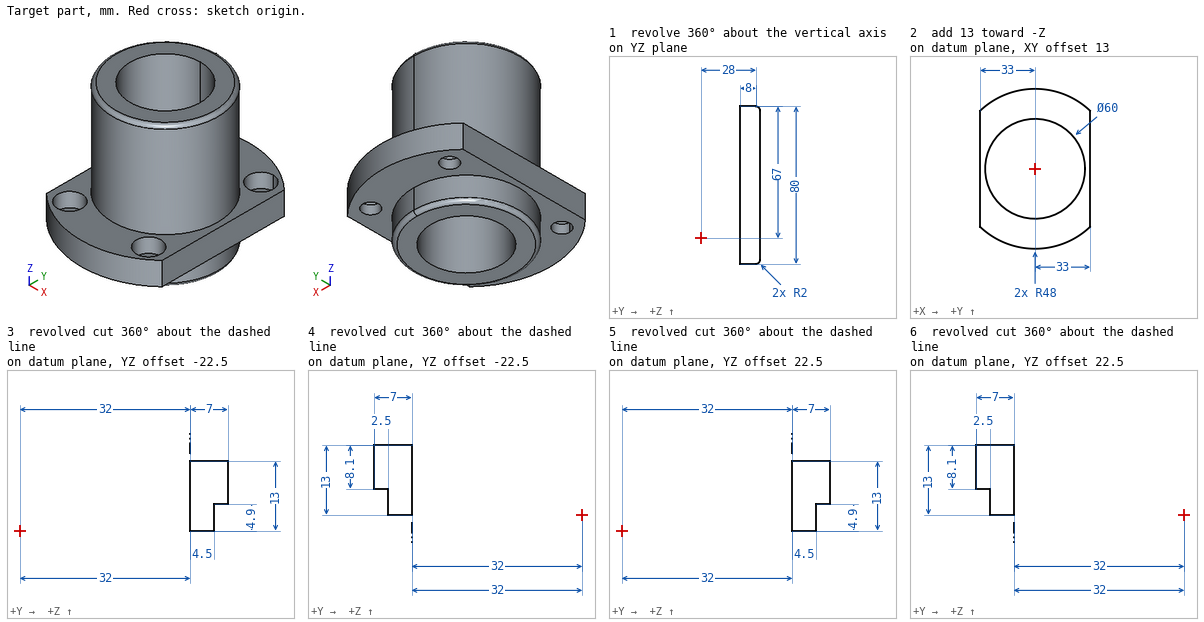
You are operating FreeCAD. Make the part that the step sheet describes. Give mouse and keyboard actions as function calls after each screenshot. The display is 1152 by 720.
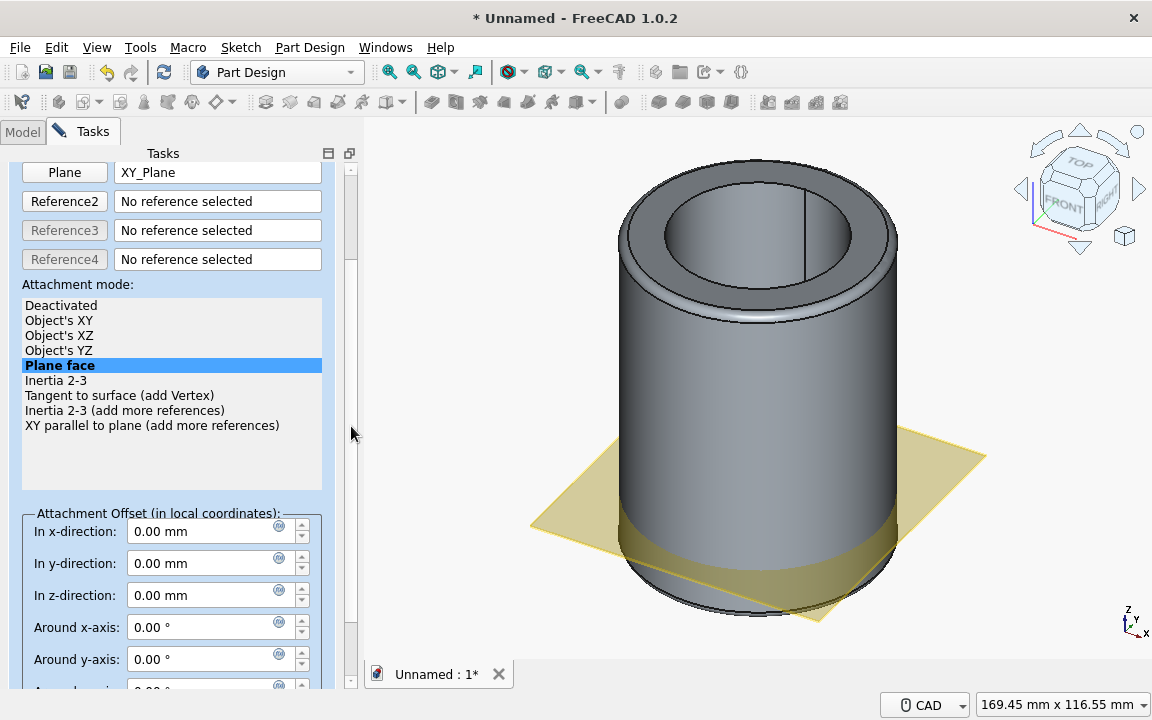
triple_click(210, 595)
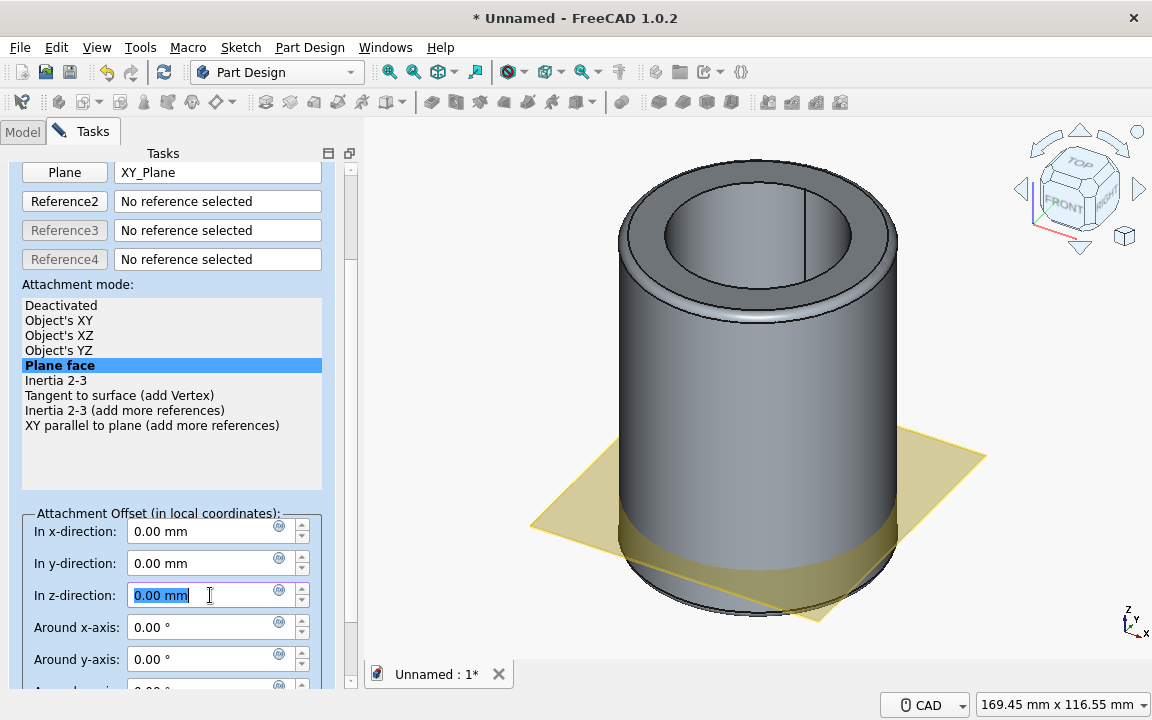
text(13)
key(Tab)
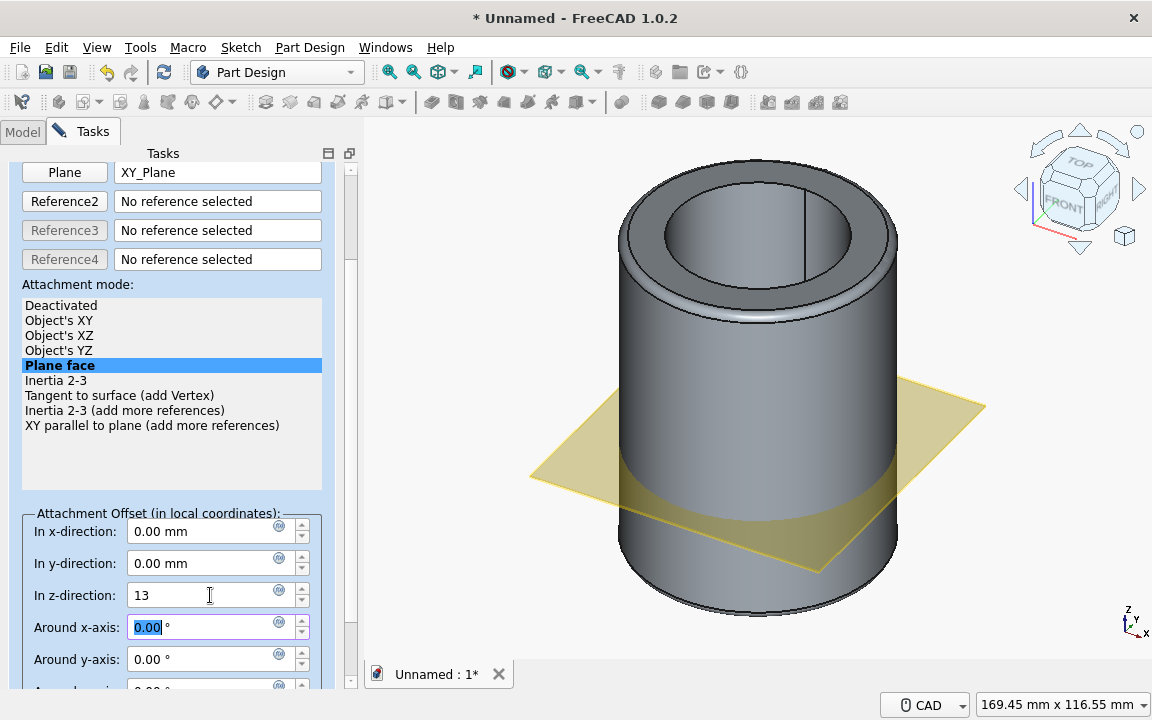
scroll(351, 426, up, 3)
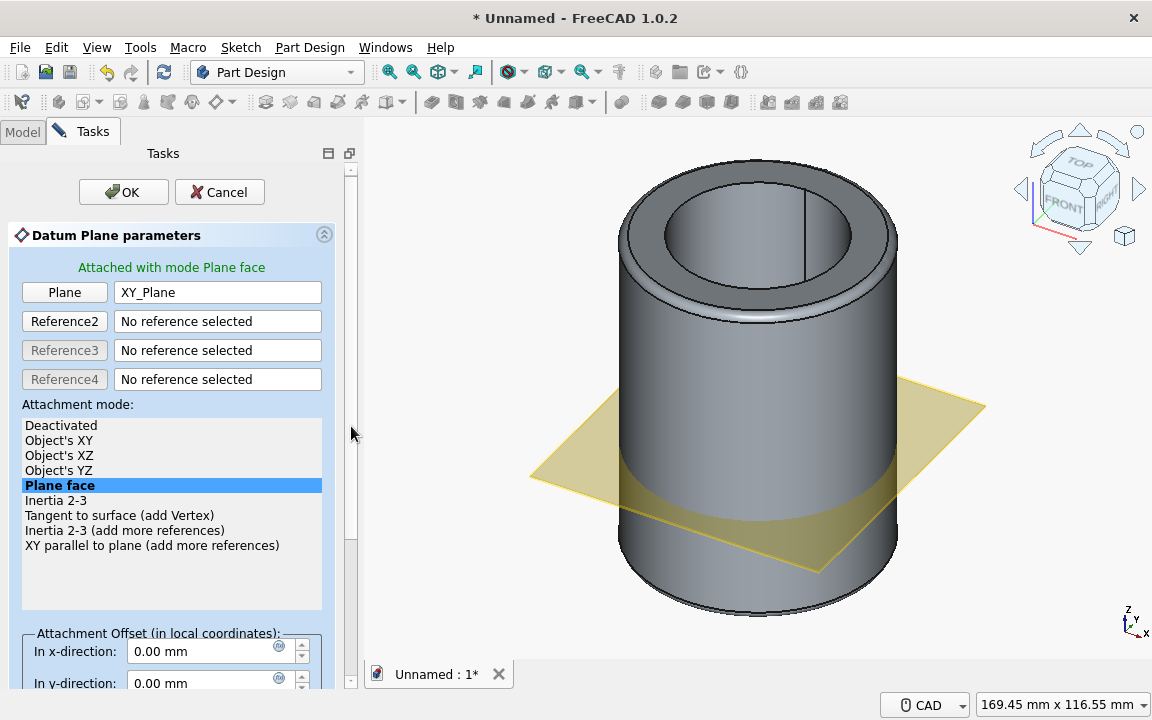
click(124, 192)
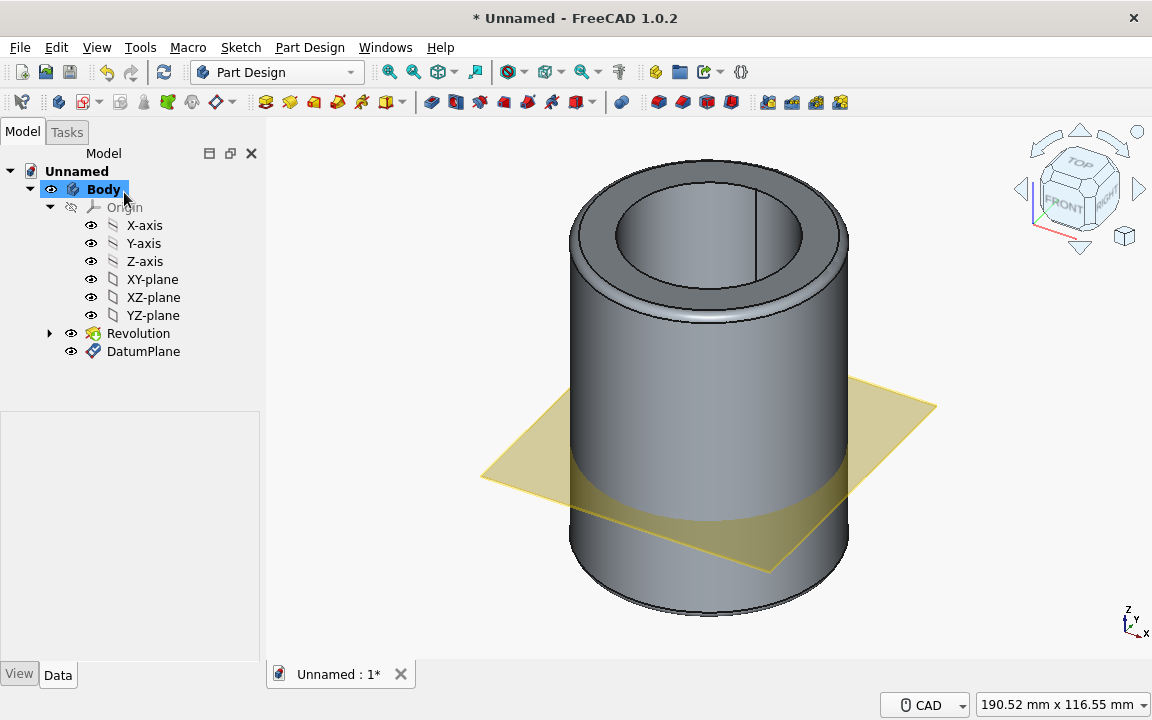
click(116, 351)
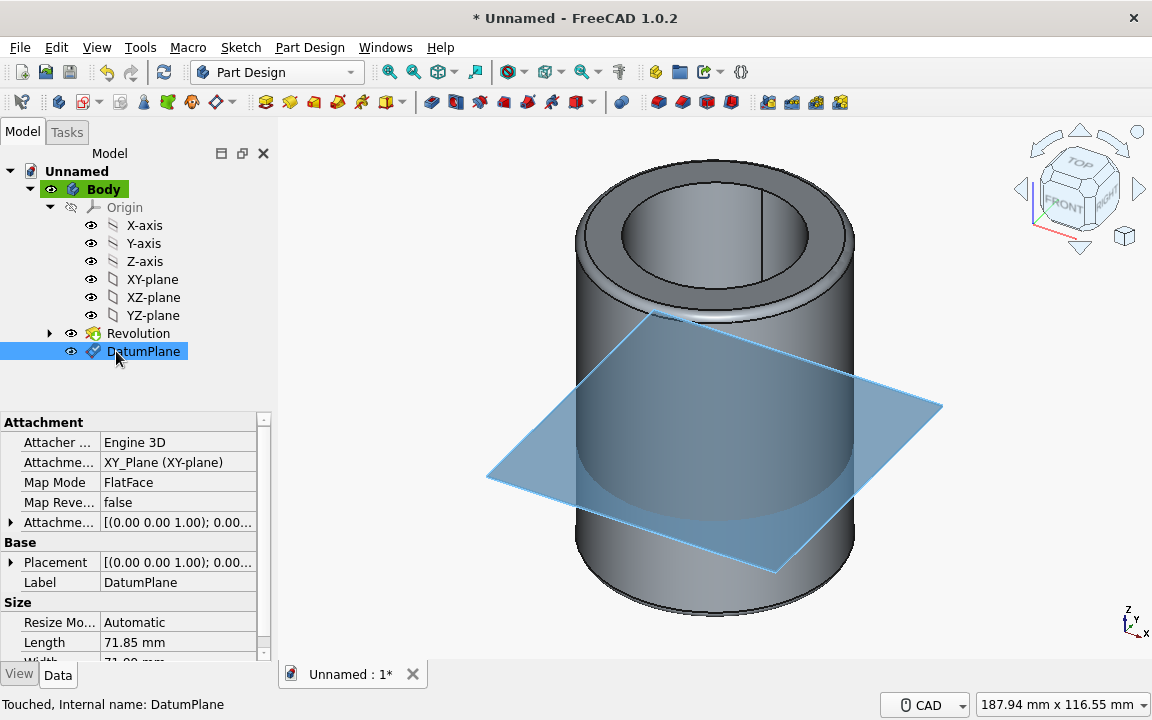
click(84, 102)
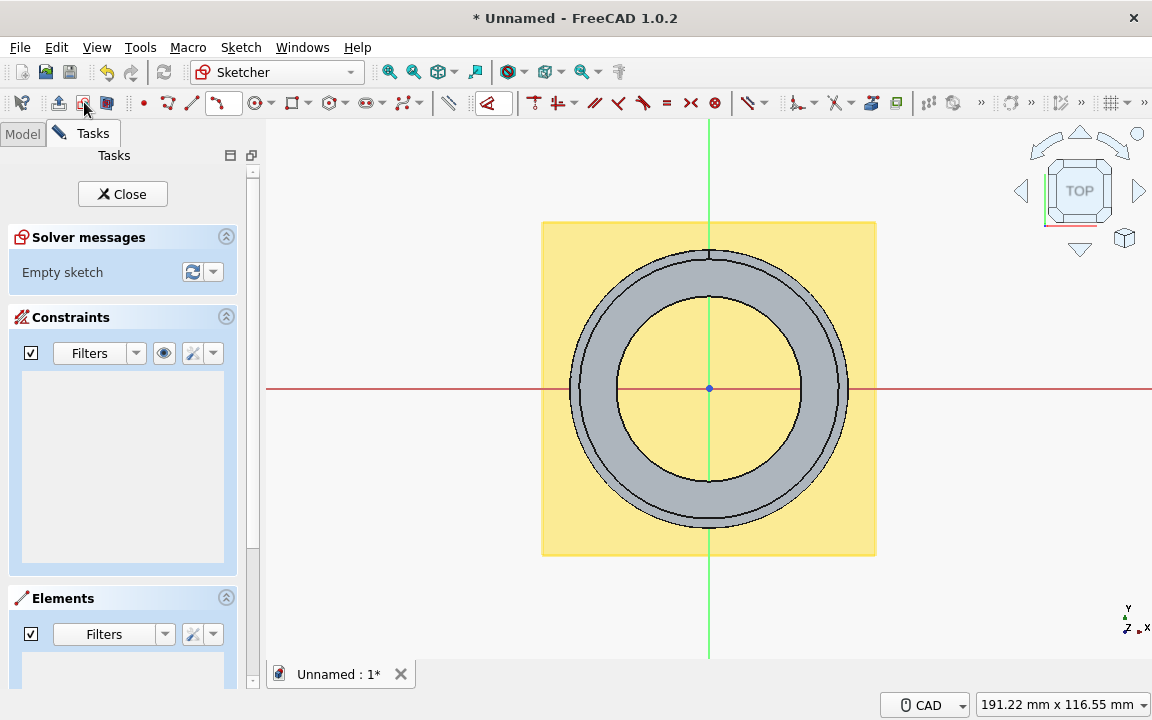
click(108, 104)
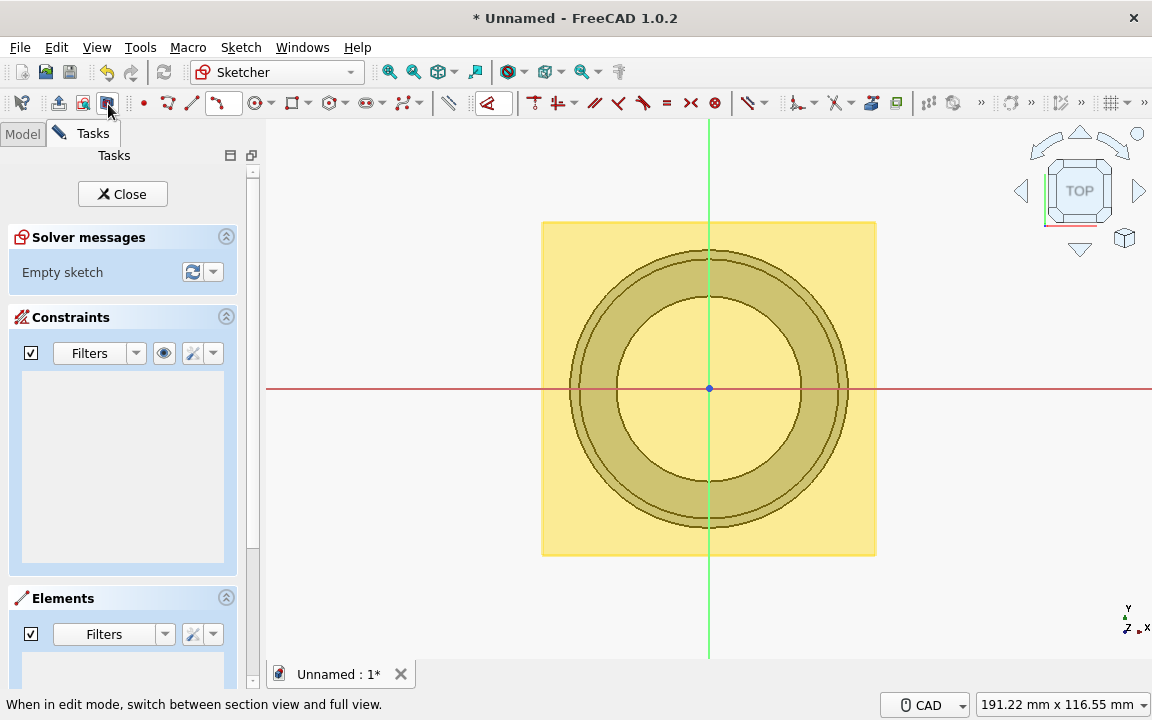
scroll(331, 389, down, 1)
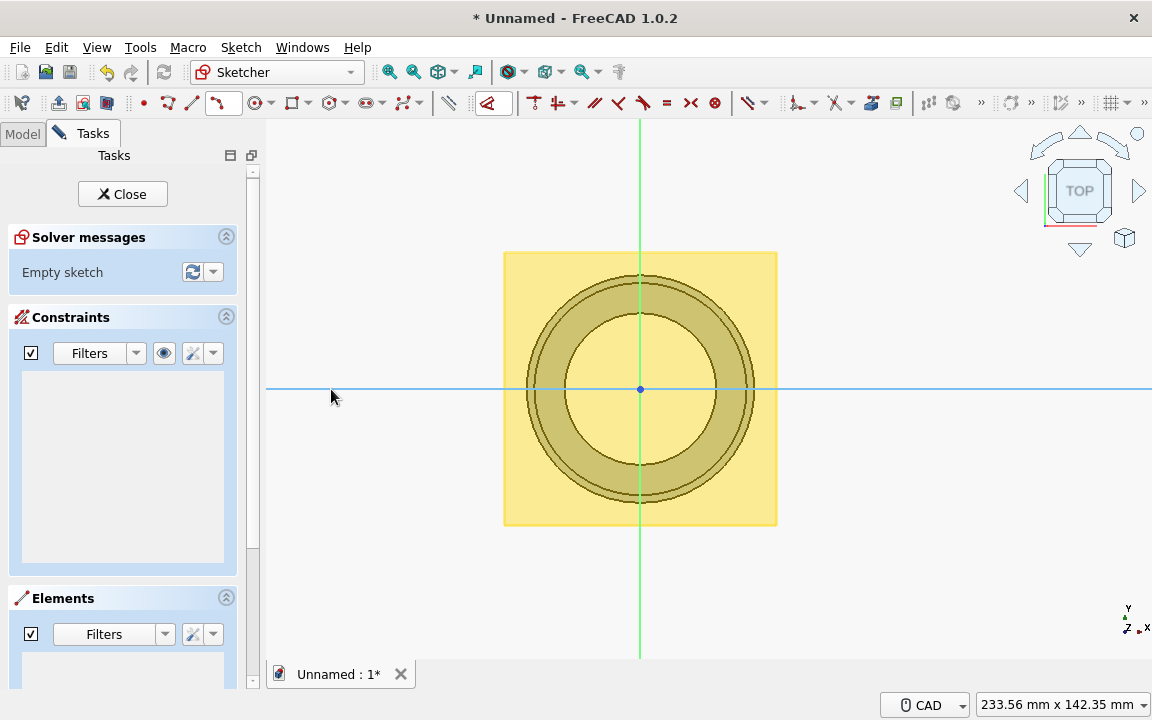
click(192, 104)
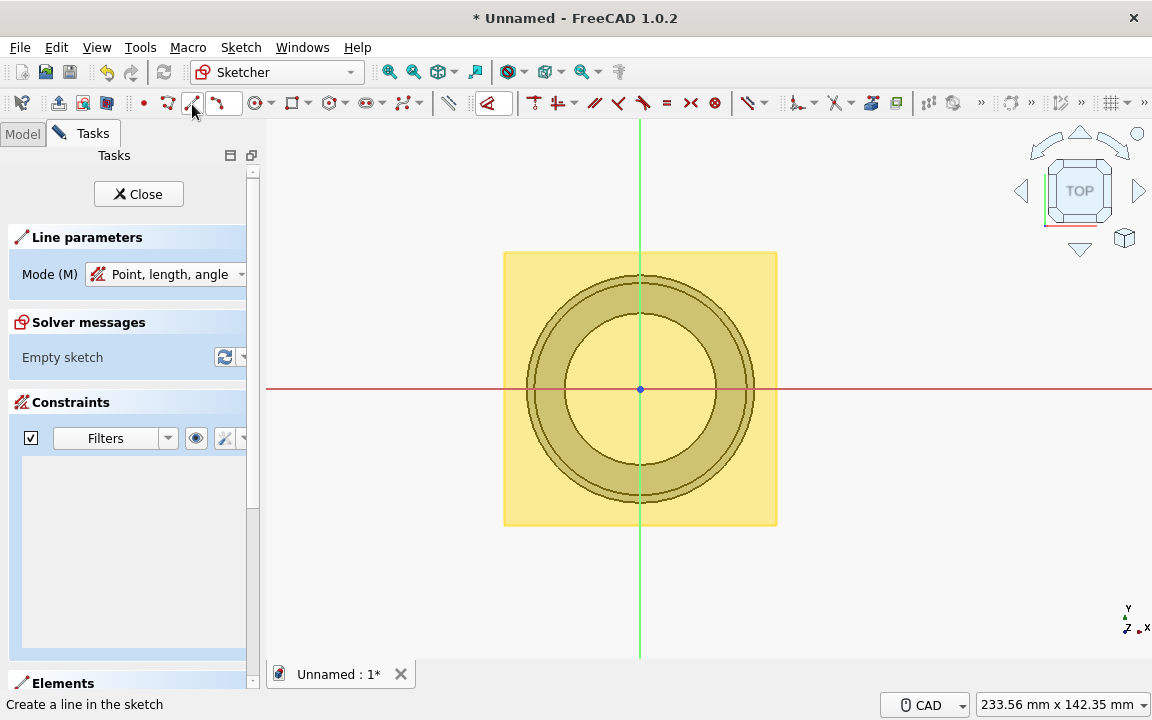
click(515, 257)
click(515, 521)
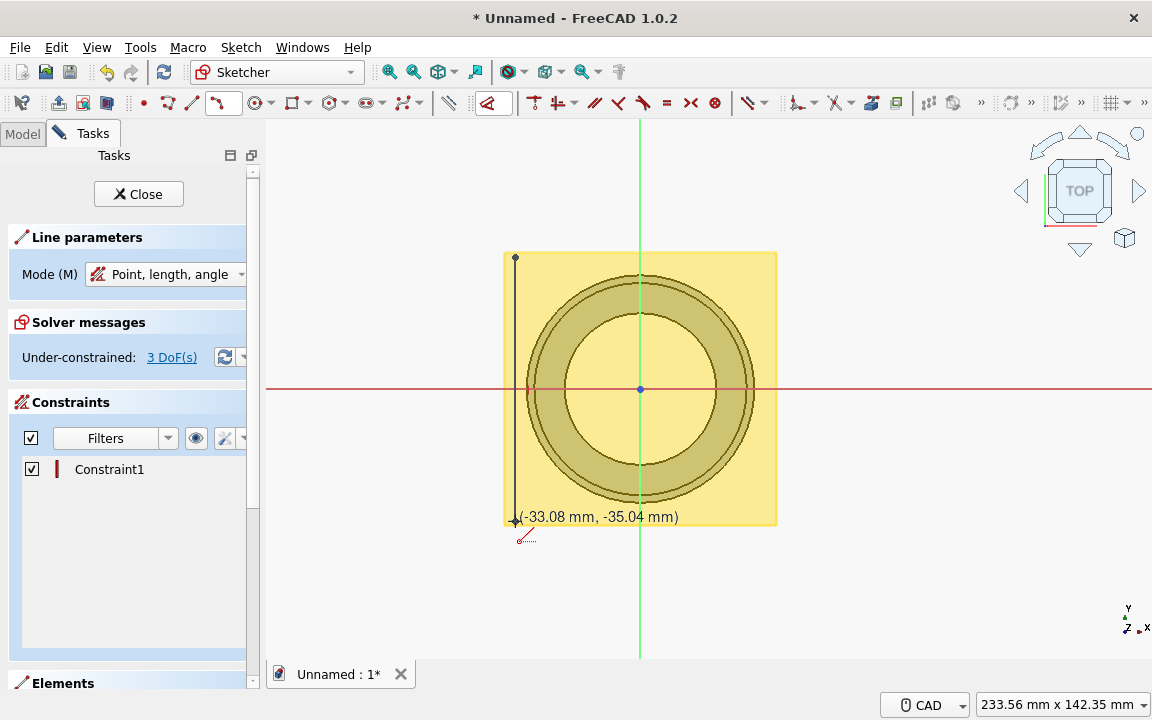
click(766, 521)
click(766, 257)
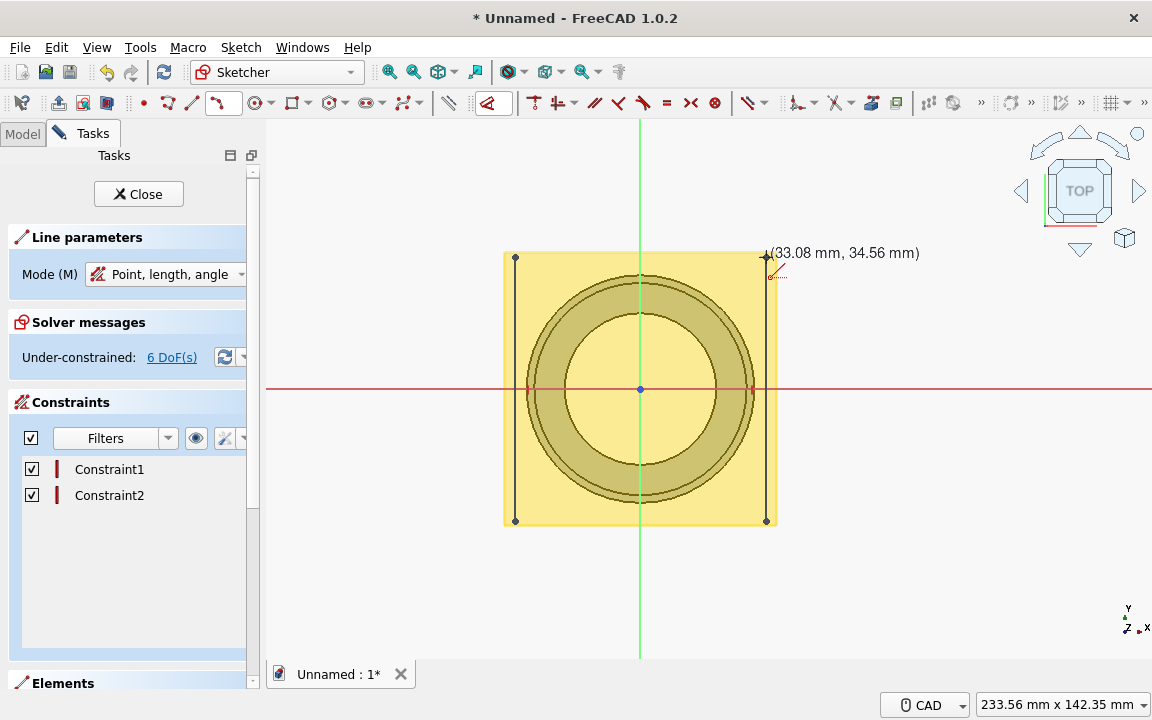
click(218, 104)